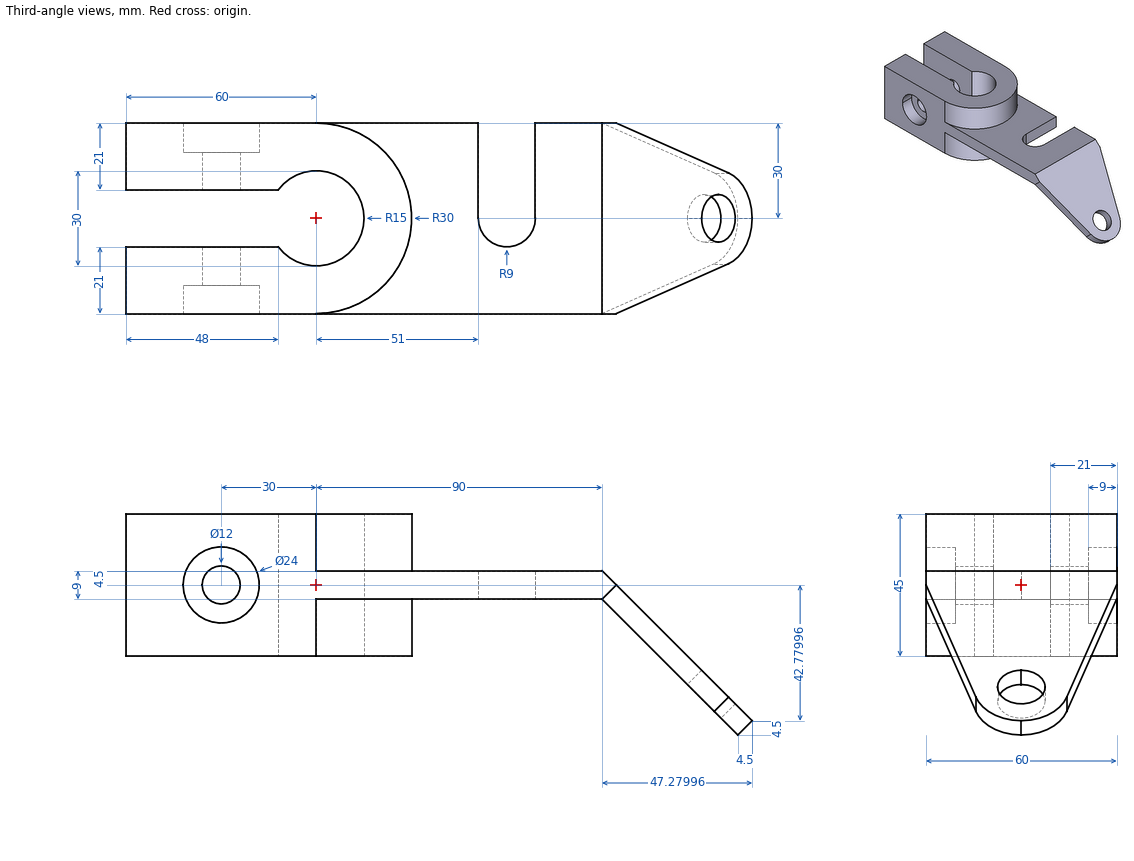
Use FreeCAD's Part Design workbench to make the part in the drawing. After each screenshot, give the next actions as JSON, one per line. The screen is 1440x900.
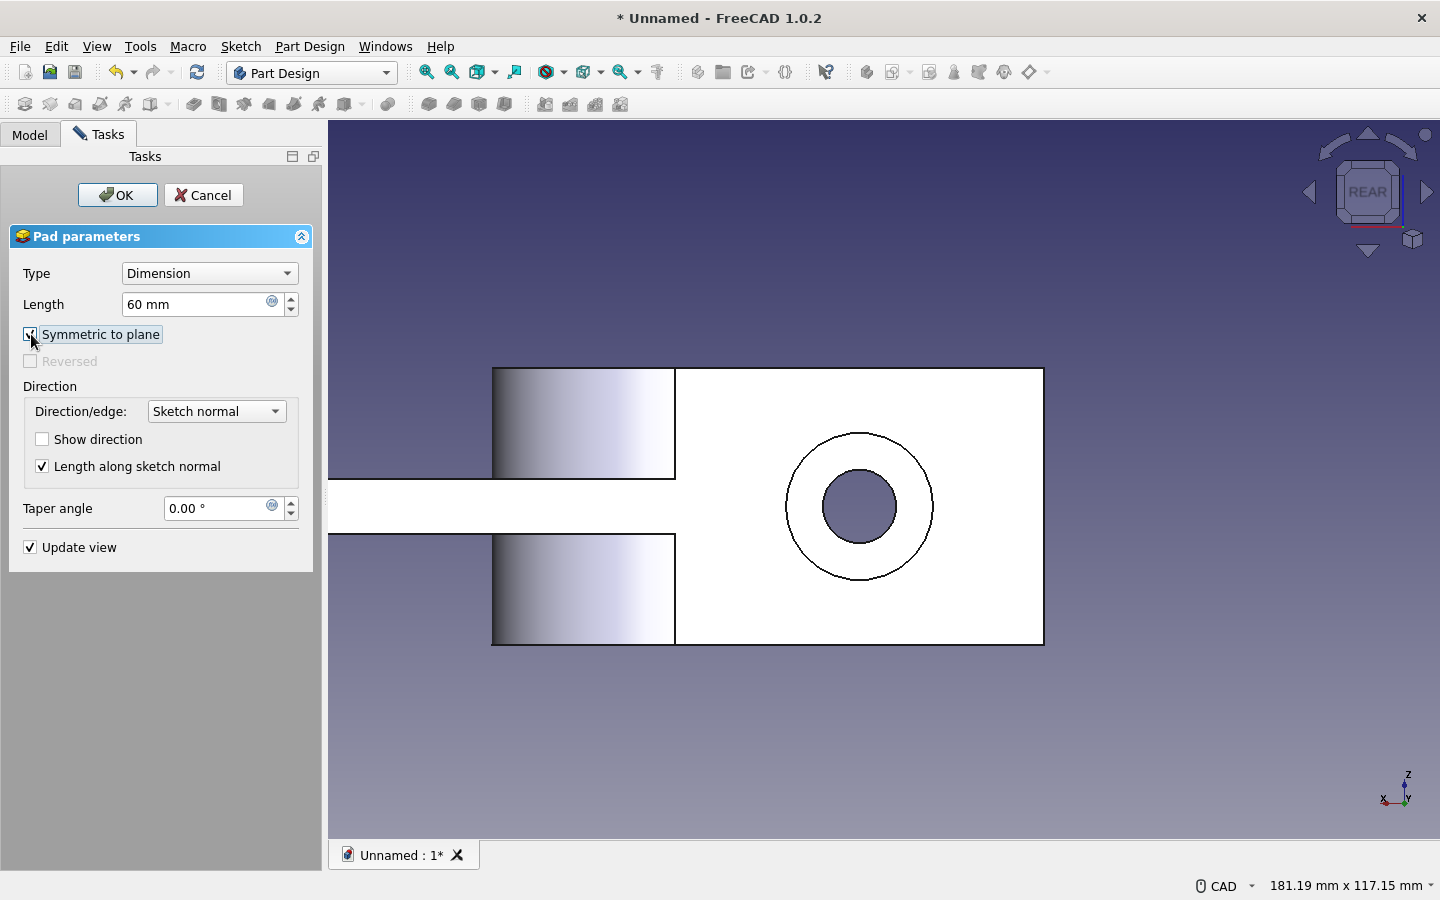
{"action": "left_click", "coordinate": [118, 195]}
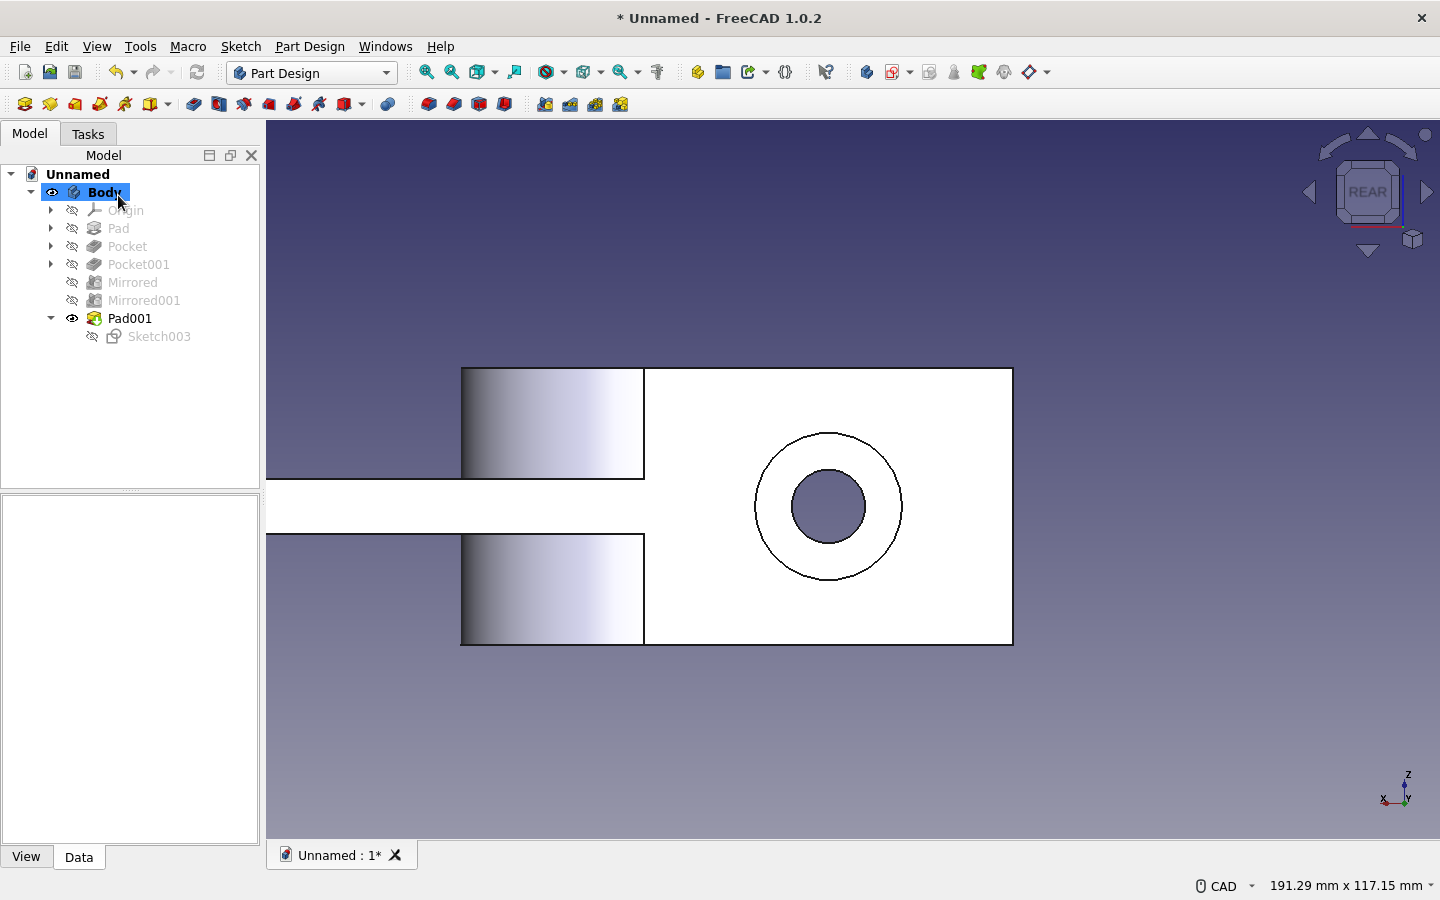
{"action": "left_click", "coordinate": [427, 72]}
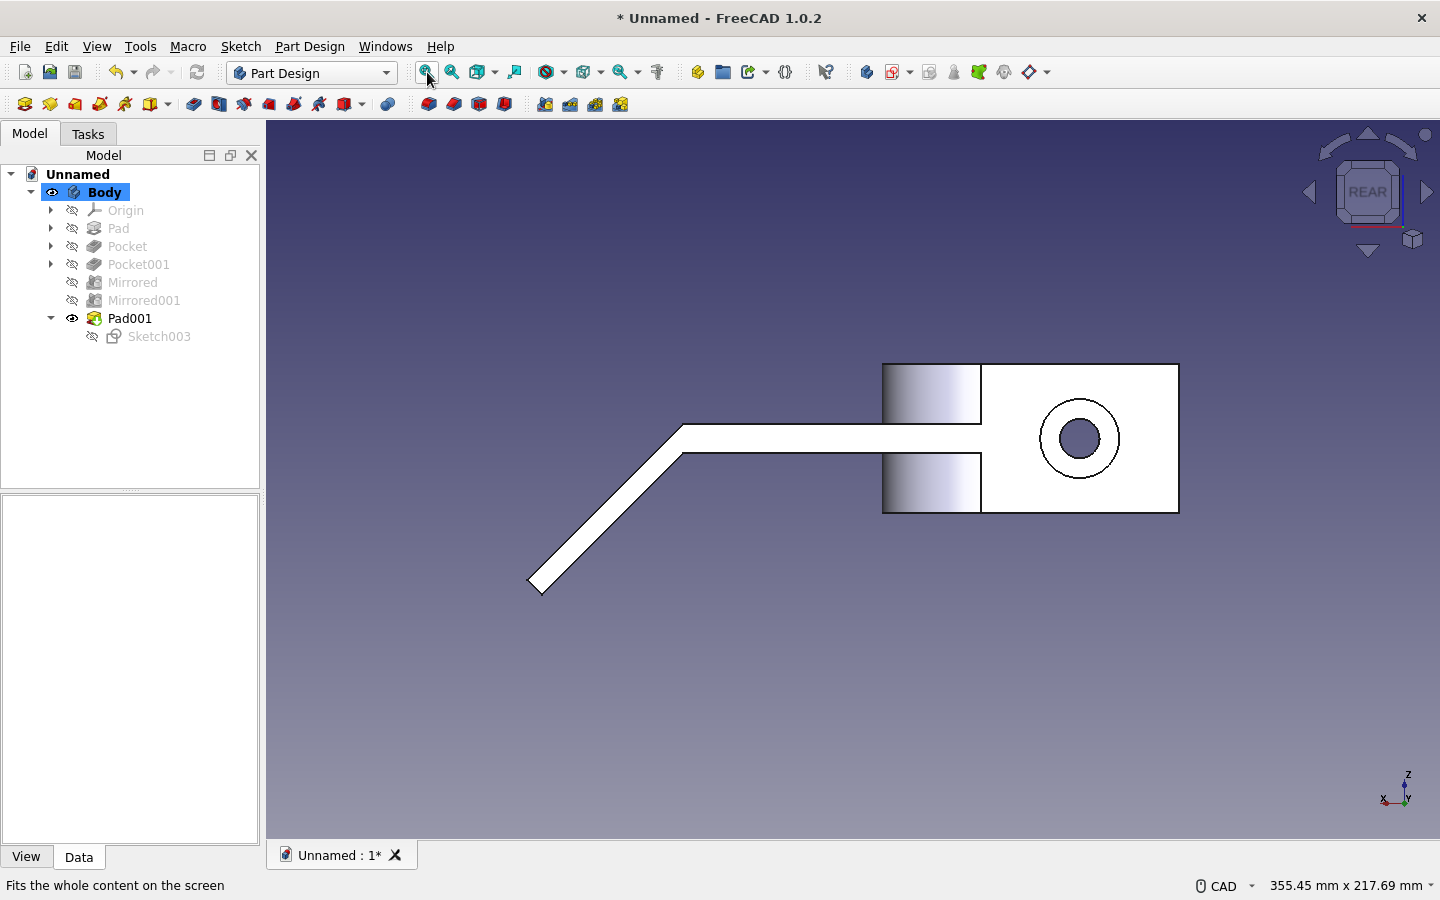
{"action": "key", "text": "5"}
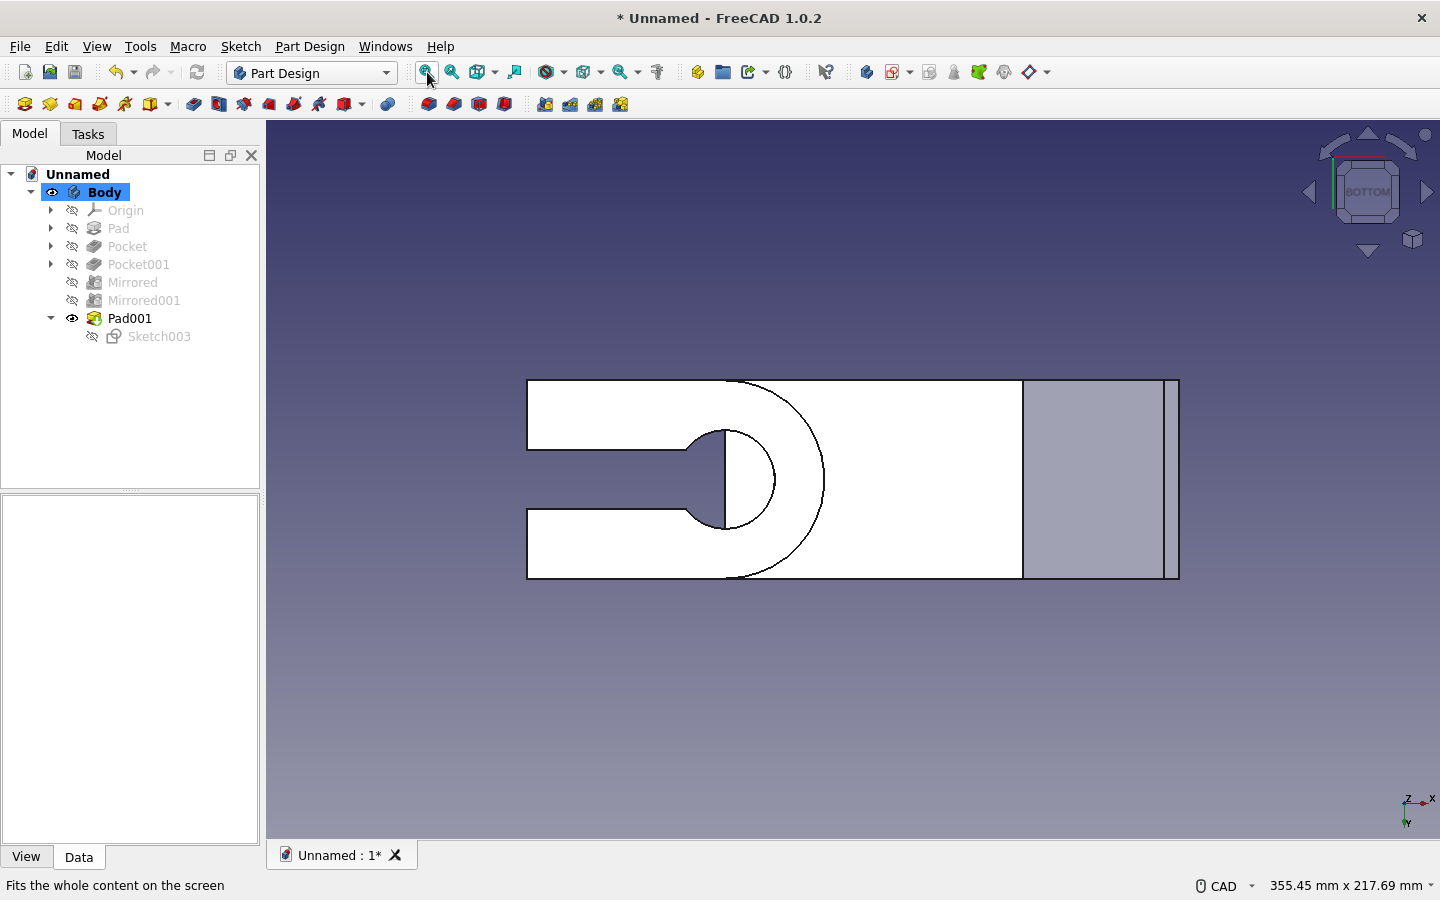
{"action": "left_click", "coordinate": [916, 478]}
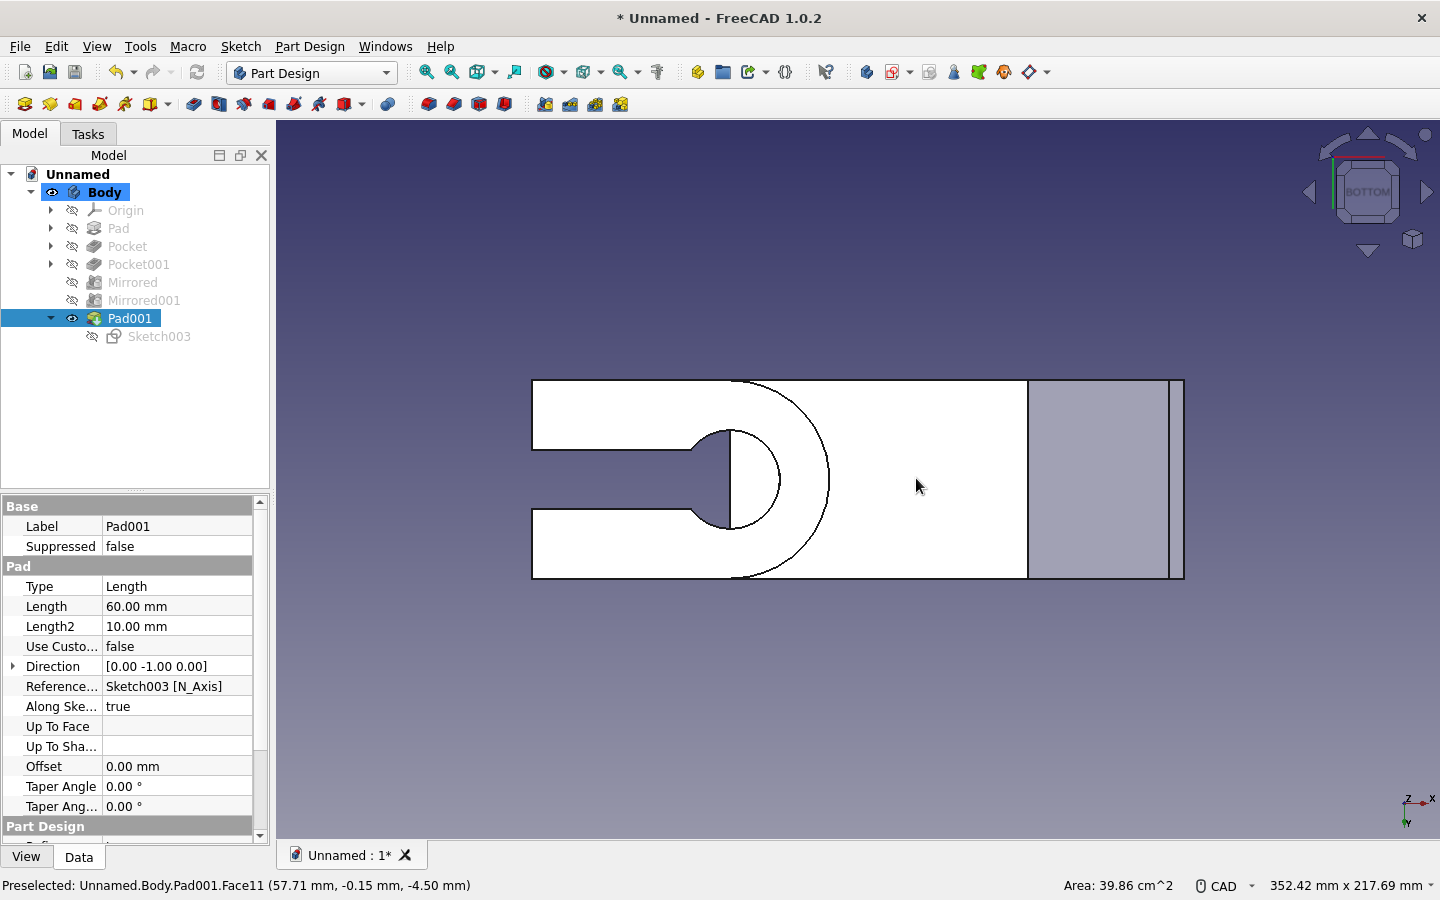
{"action": "left_click", "coordinate": [892, 72]}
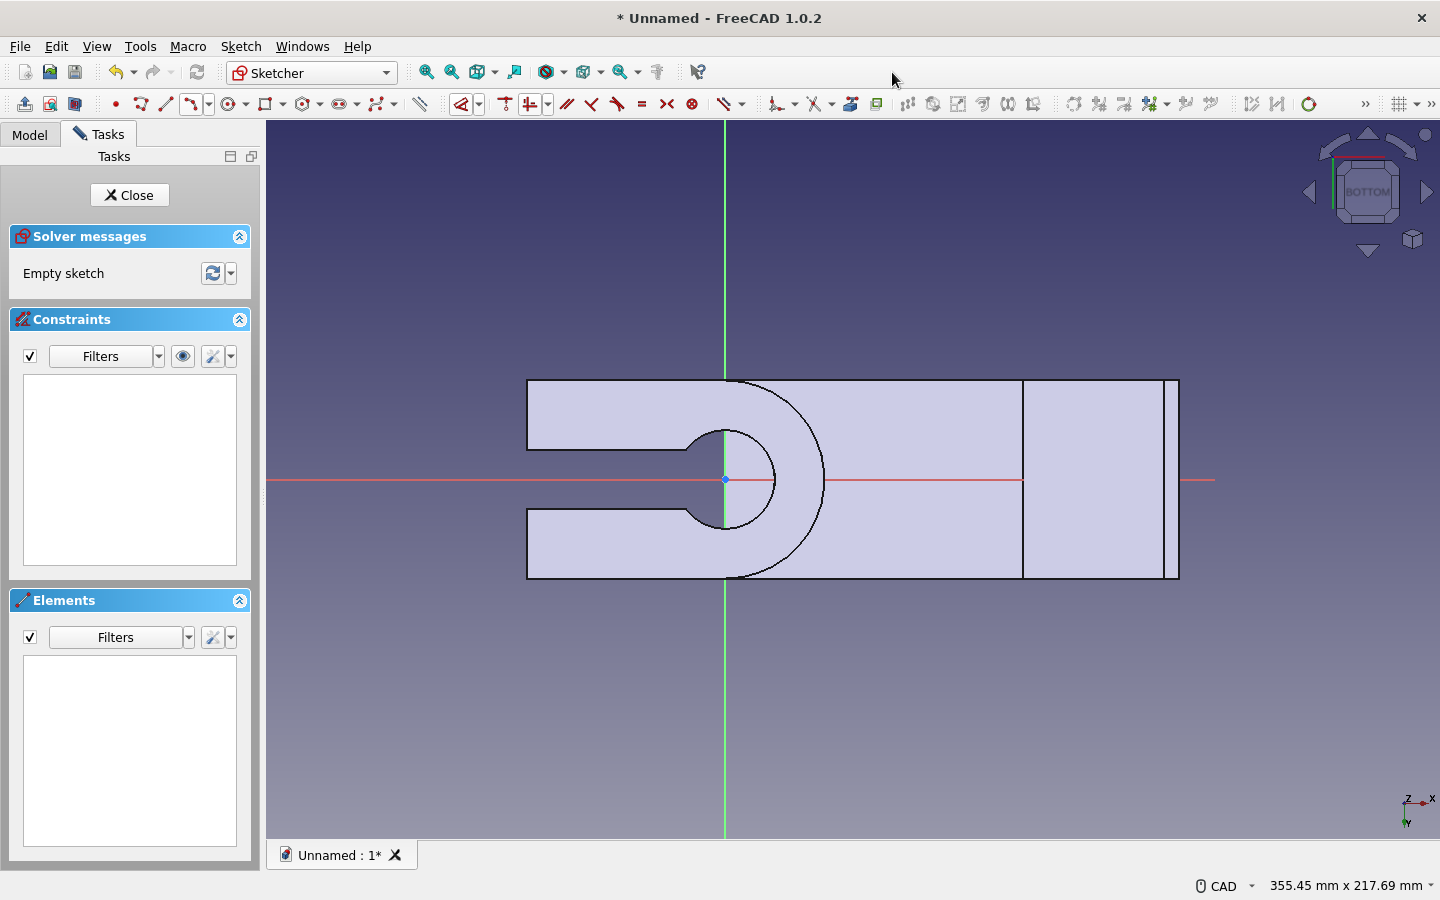
{"action": "scroll", "coordinate": [863, 529], "scroll_direction": "up", "scroll_amount": 6}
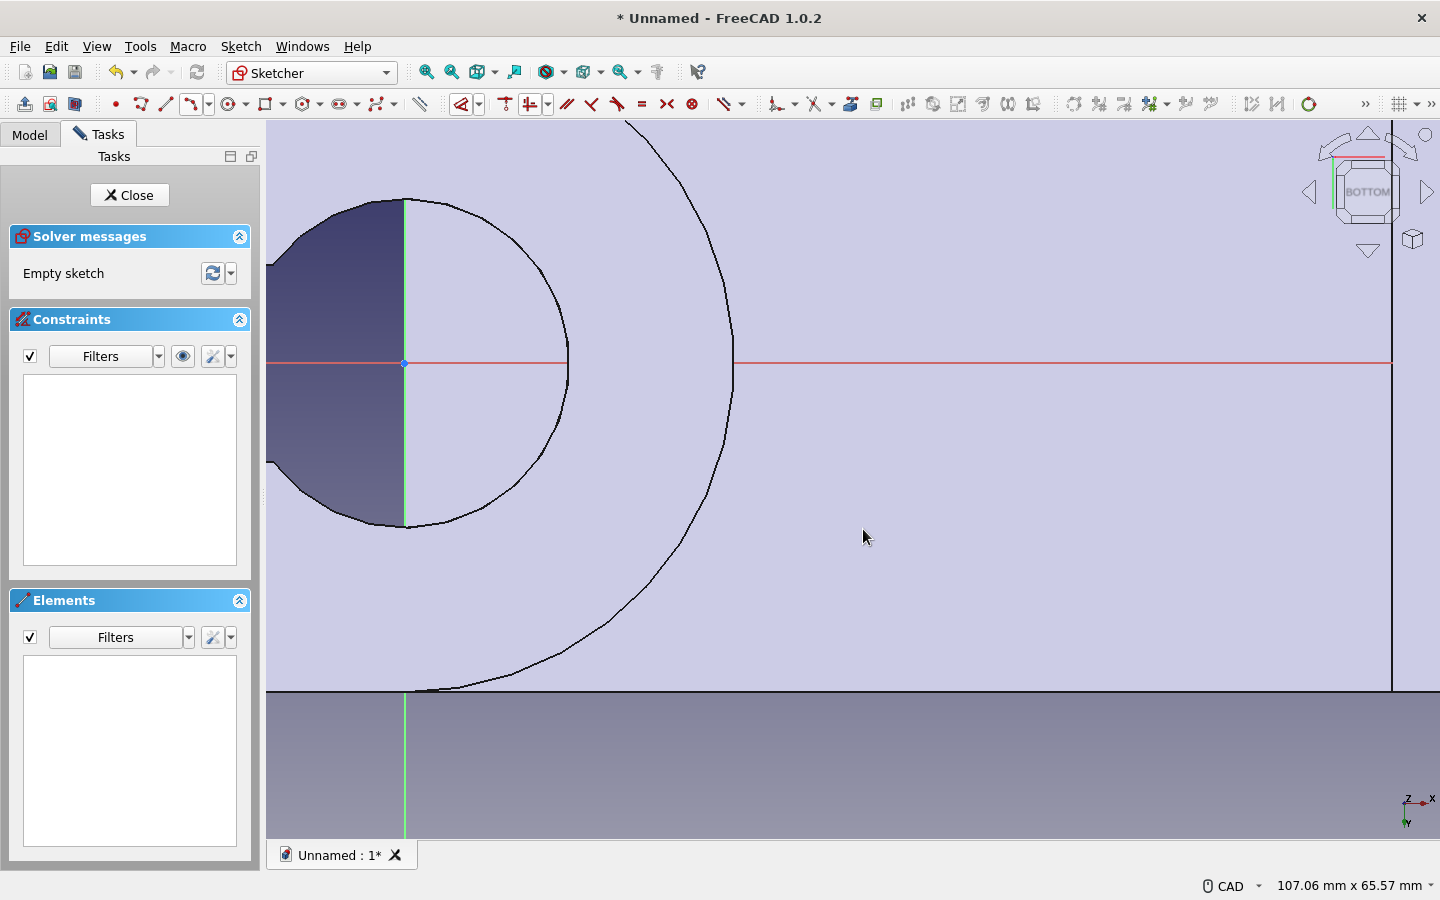
{"action": "left_click", "coordinate": [141, 104]}